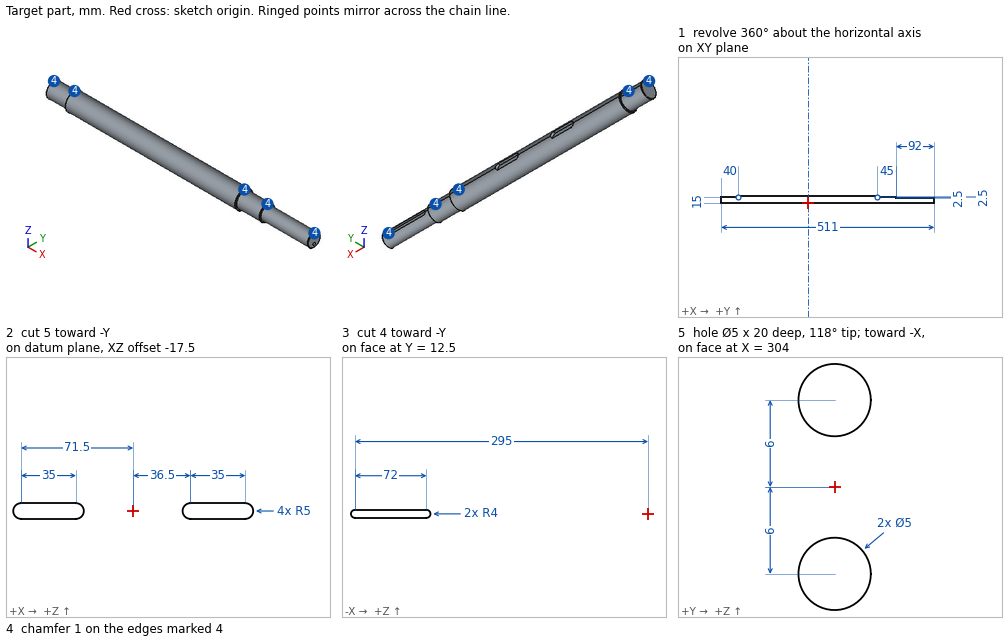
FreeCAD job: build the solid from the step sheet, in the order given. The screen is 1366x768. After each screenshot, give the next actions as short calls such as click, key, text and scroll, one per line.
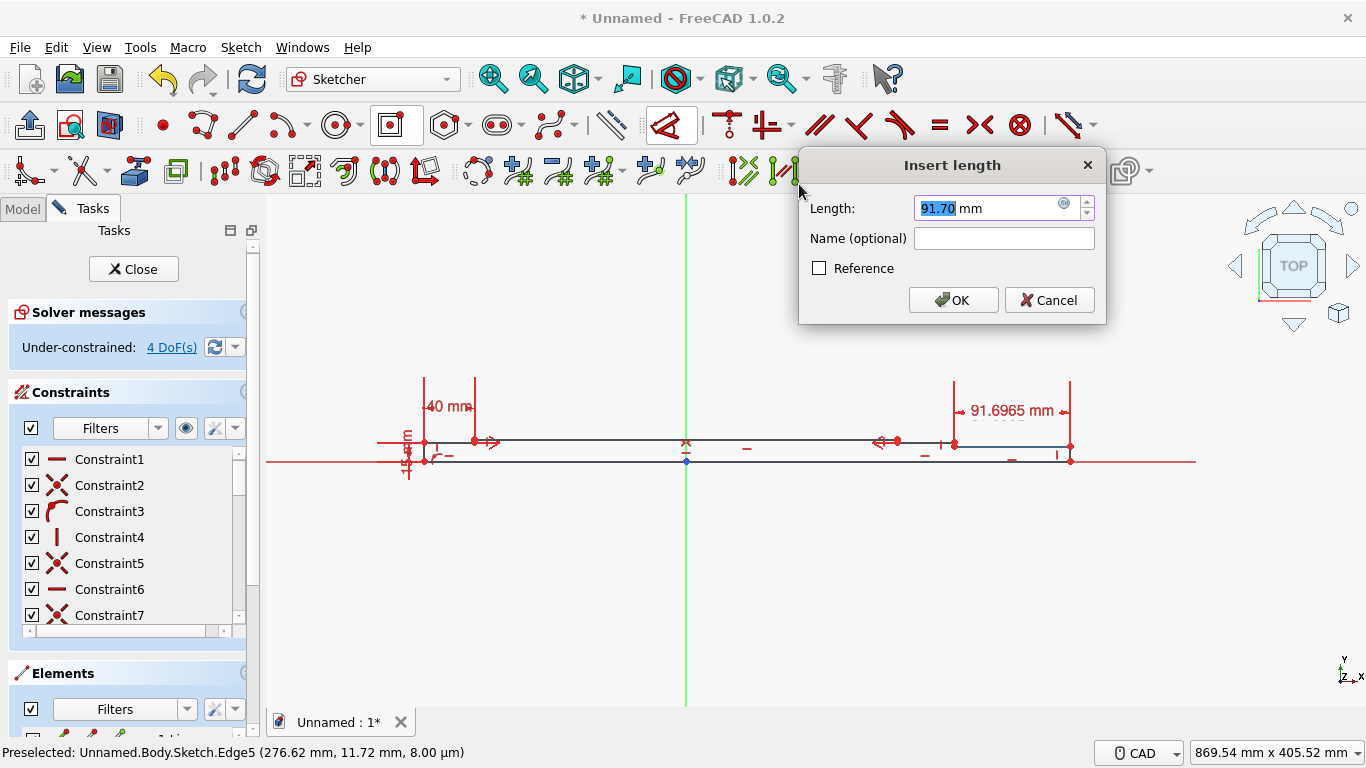
text(92)
key(Return)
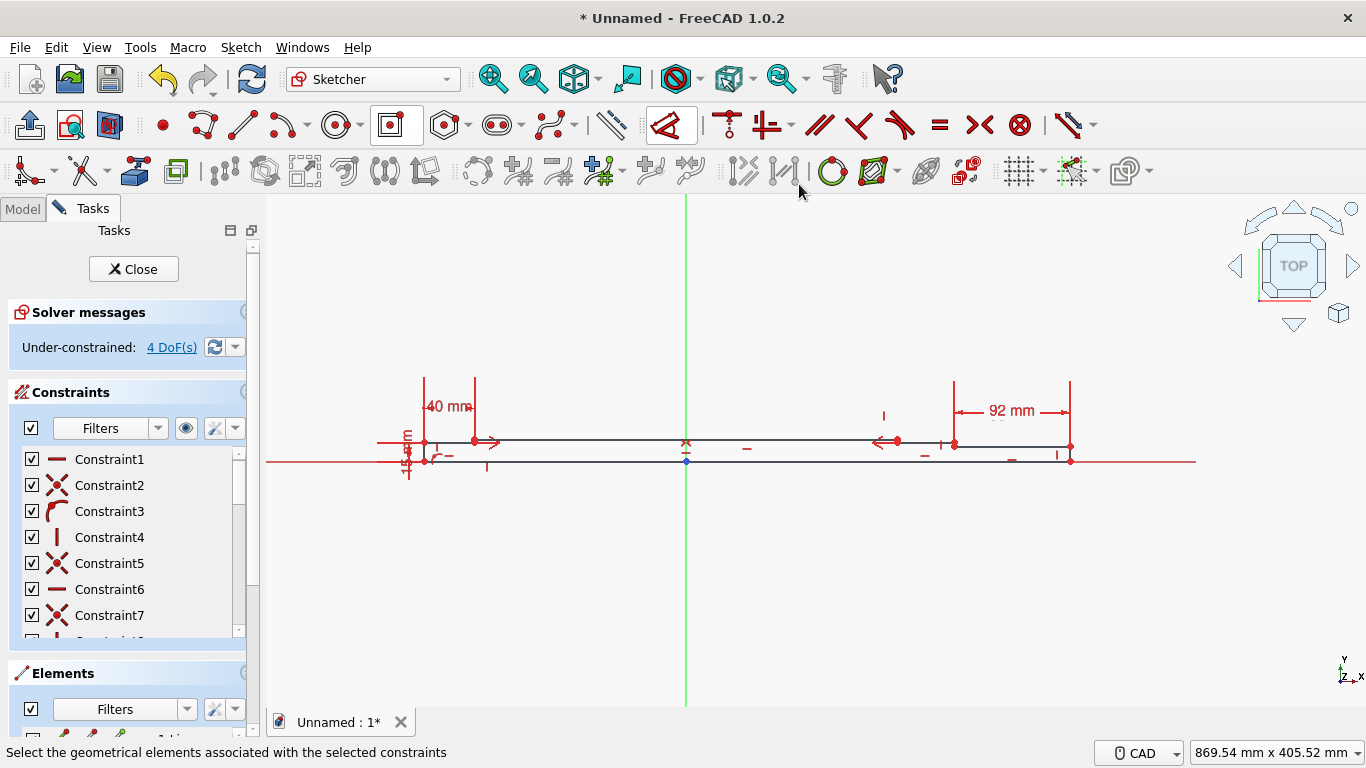
click(914, 443)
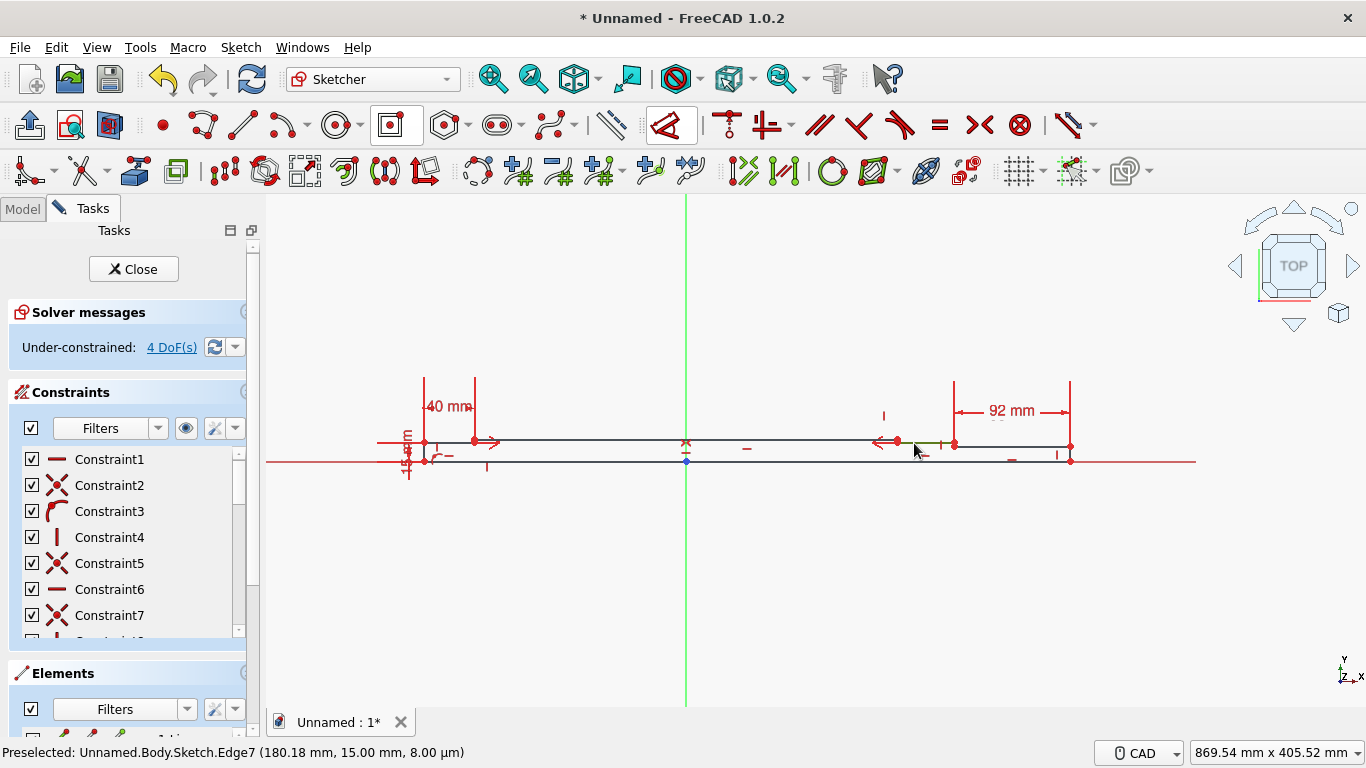
key(l)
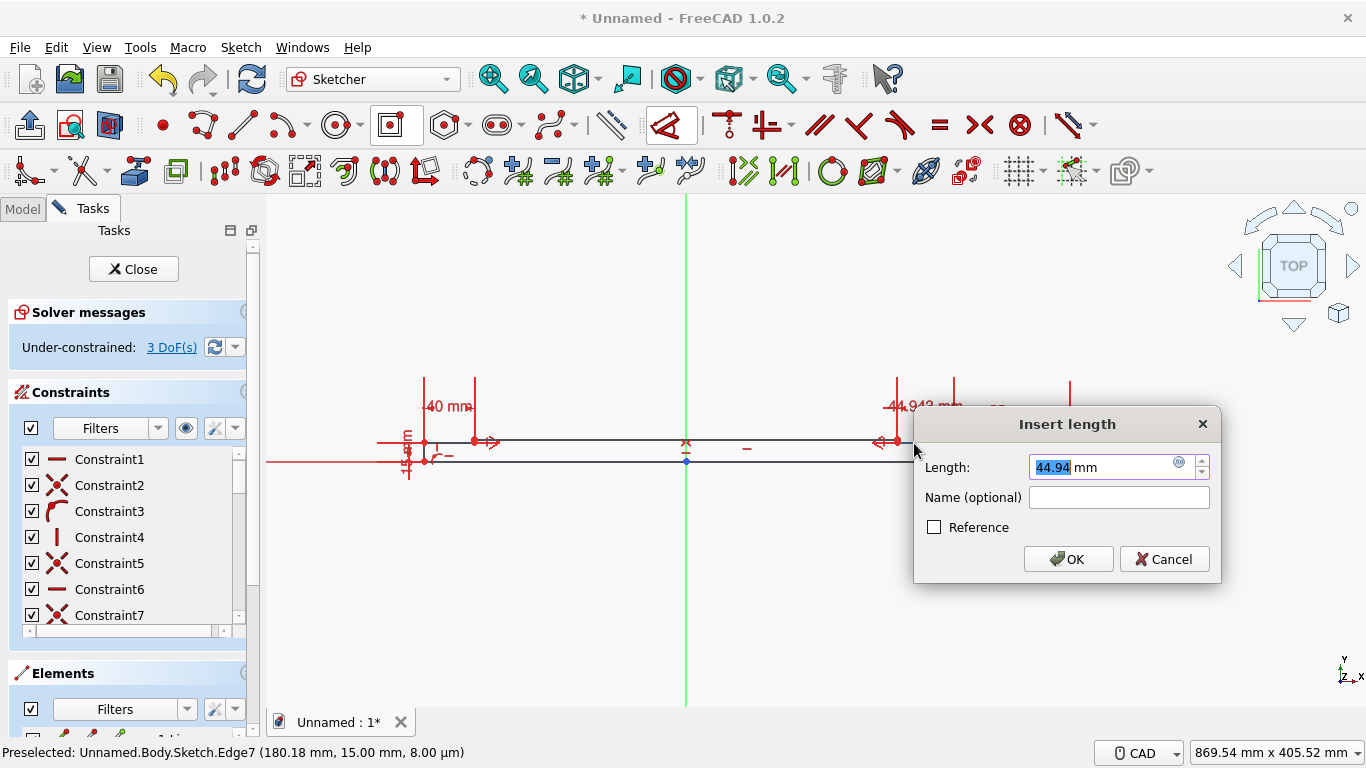
text(45)
key(Return)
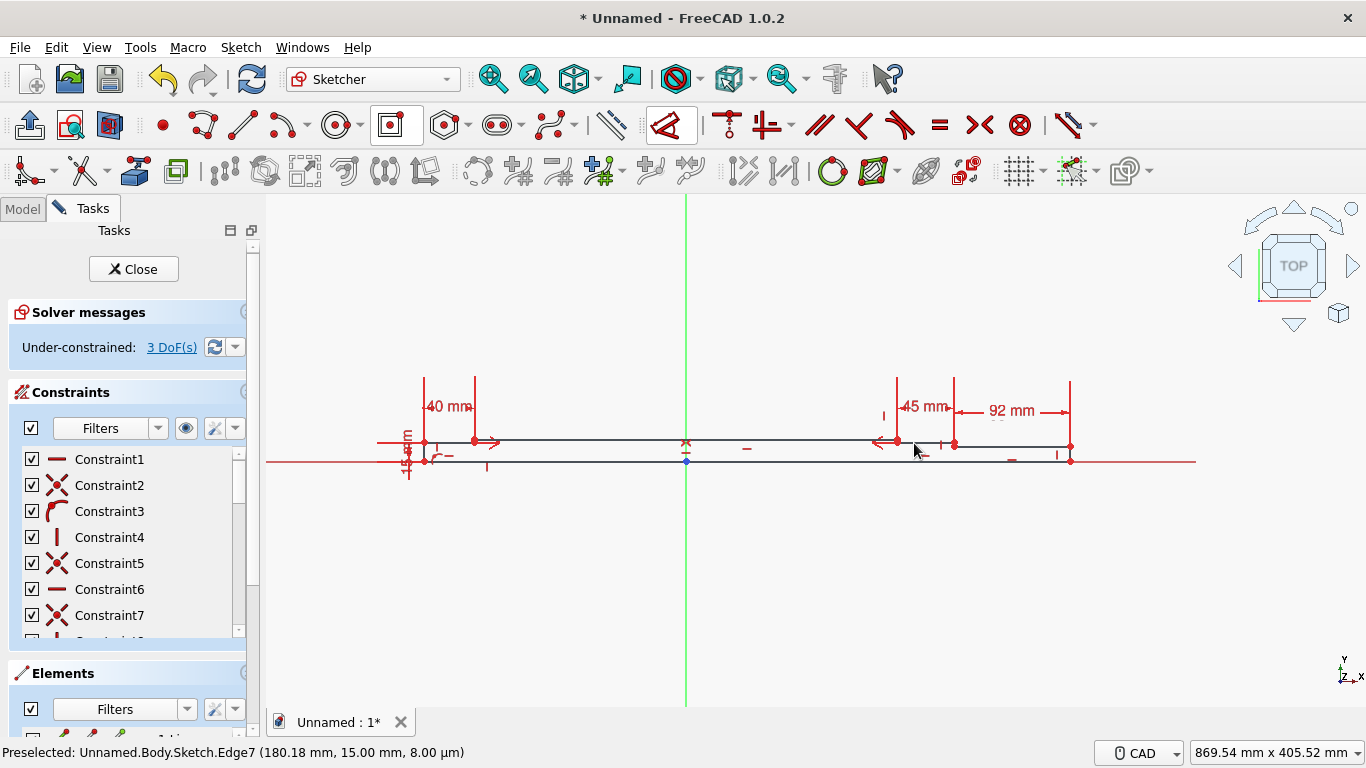
click(618, 462)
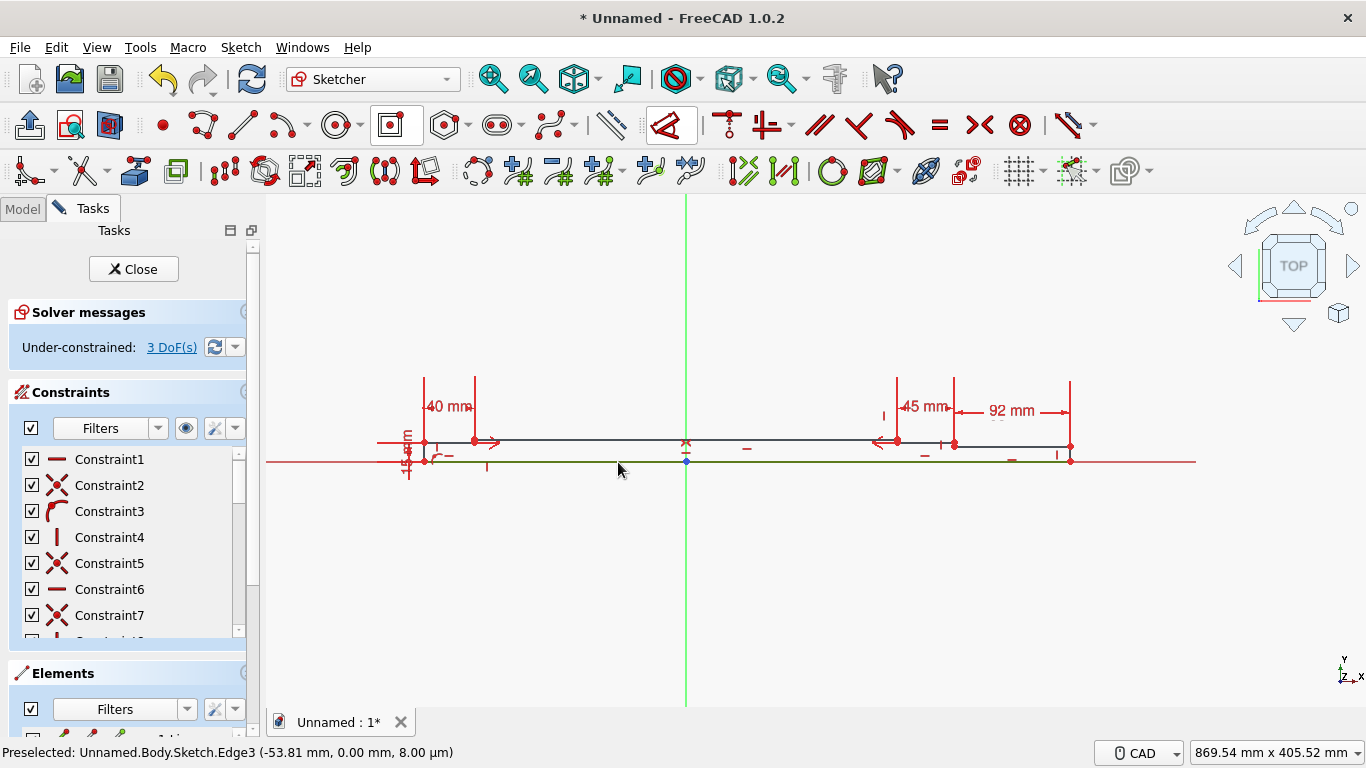
key(l)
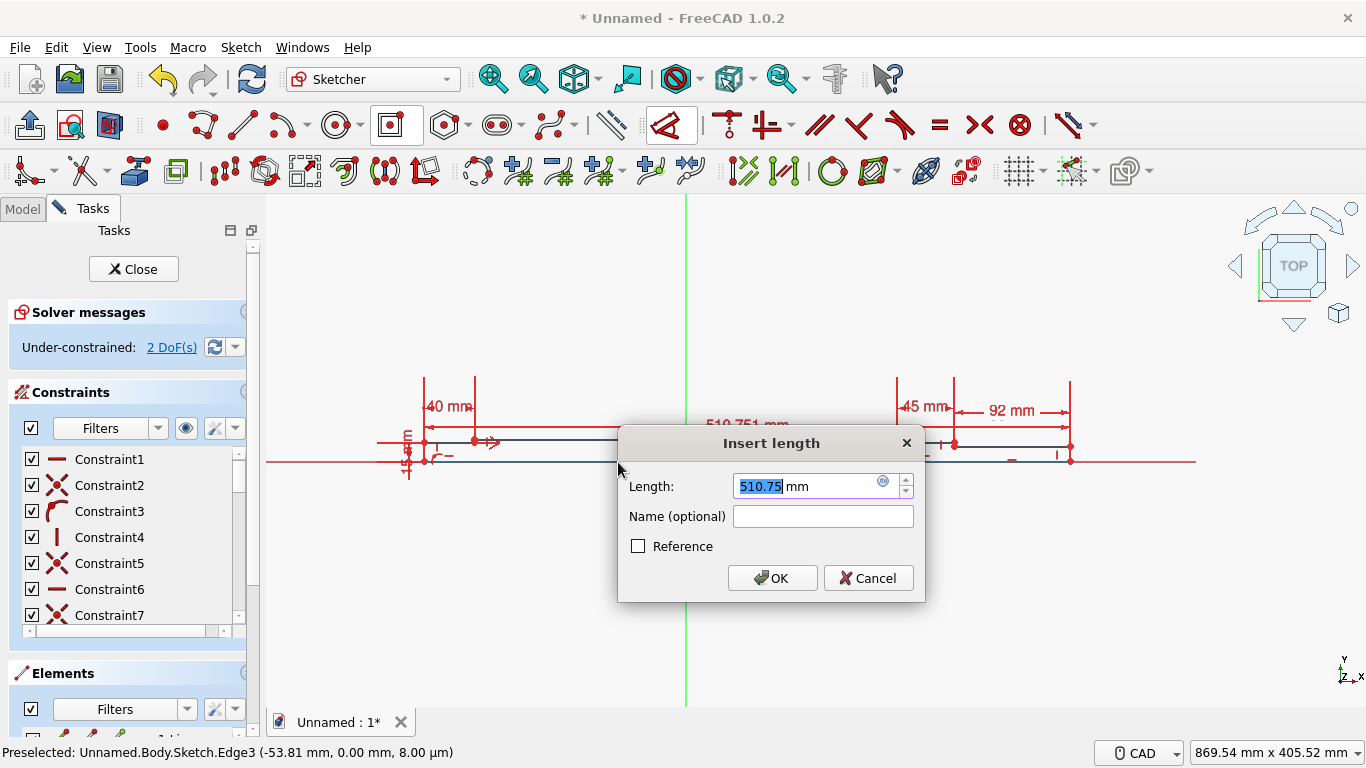
text(511)
key(Return)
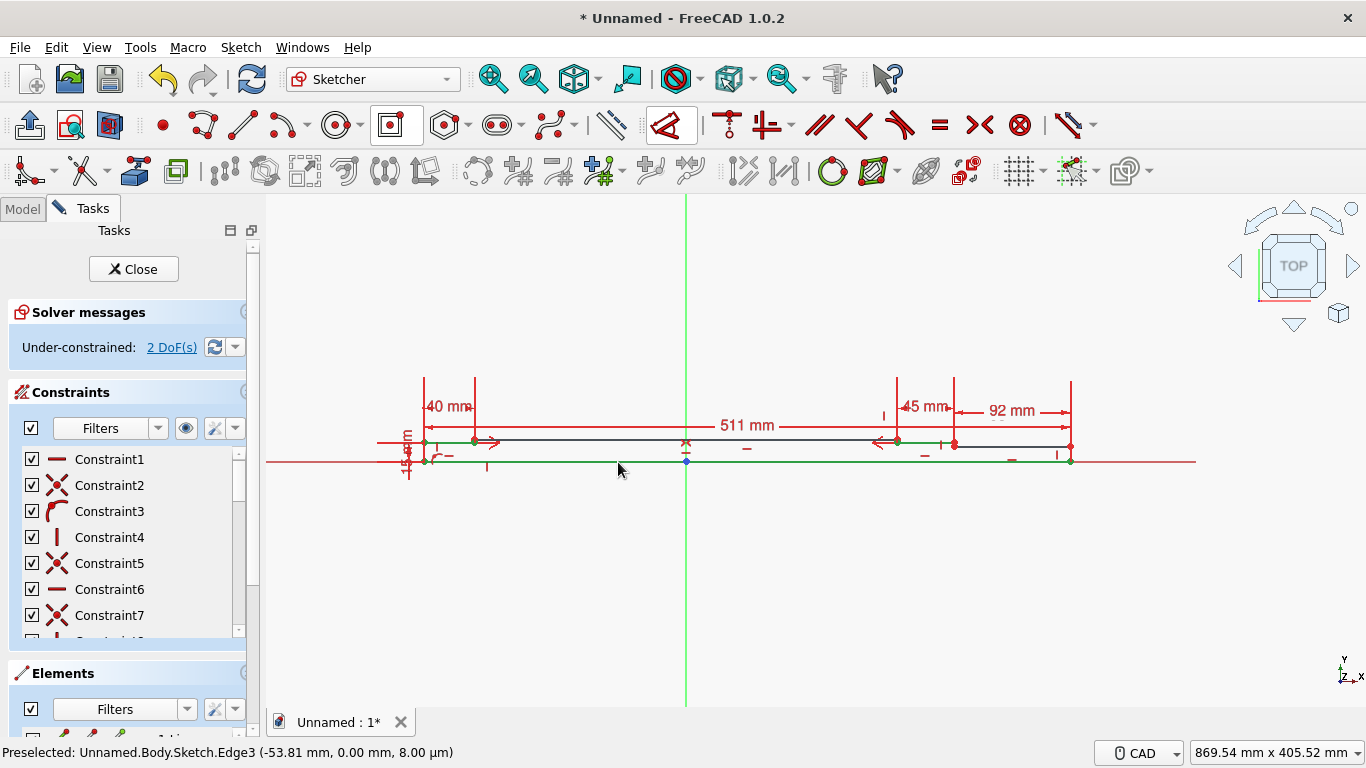
scroll(954, 445, up, 13)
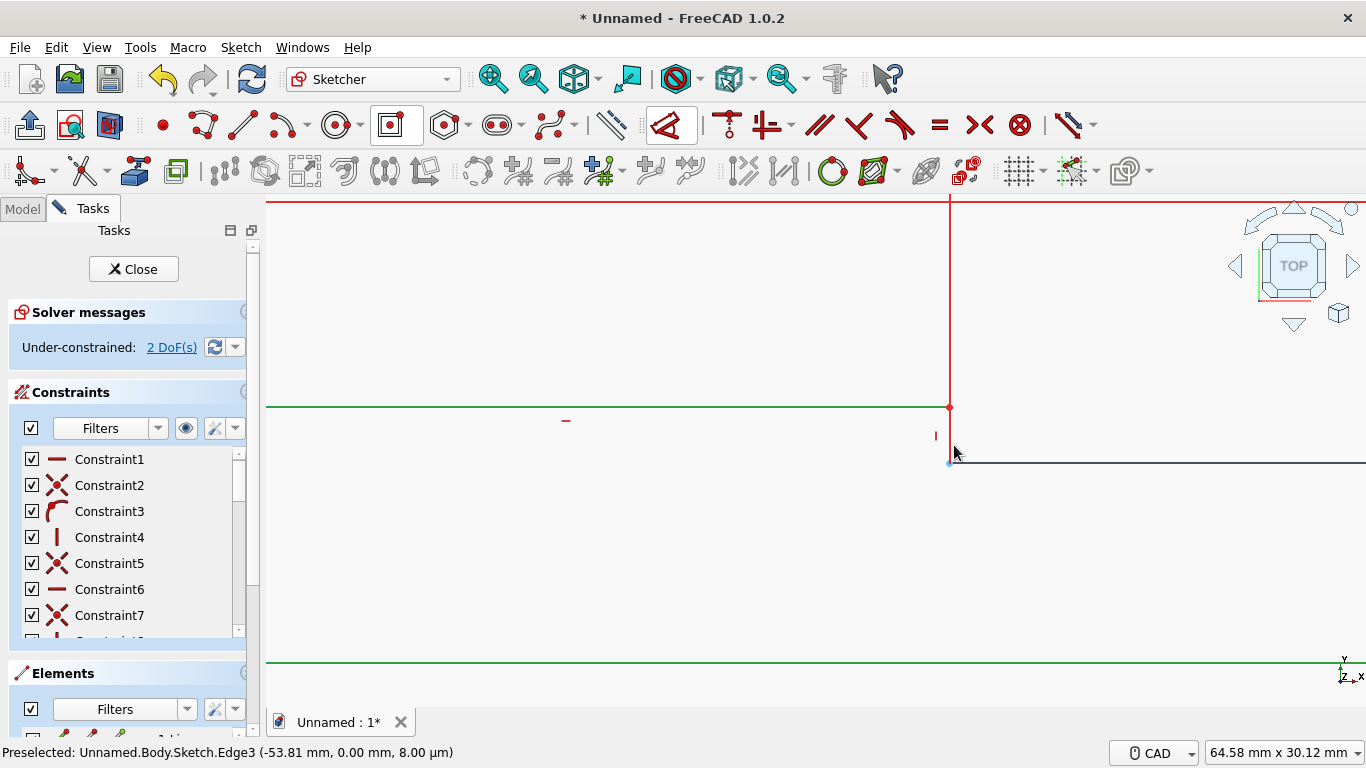
click(950, 435)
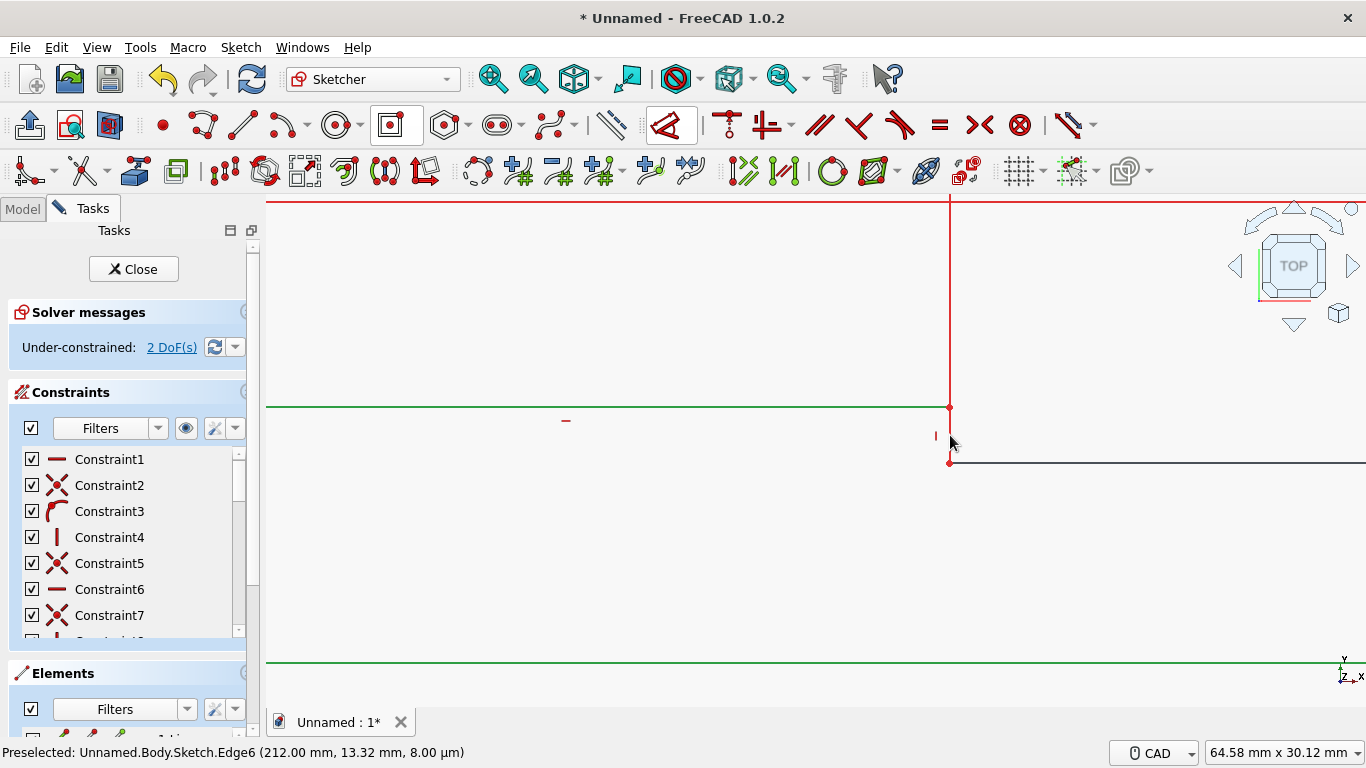
click(692, 126)